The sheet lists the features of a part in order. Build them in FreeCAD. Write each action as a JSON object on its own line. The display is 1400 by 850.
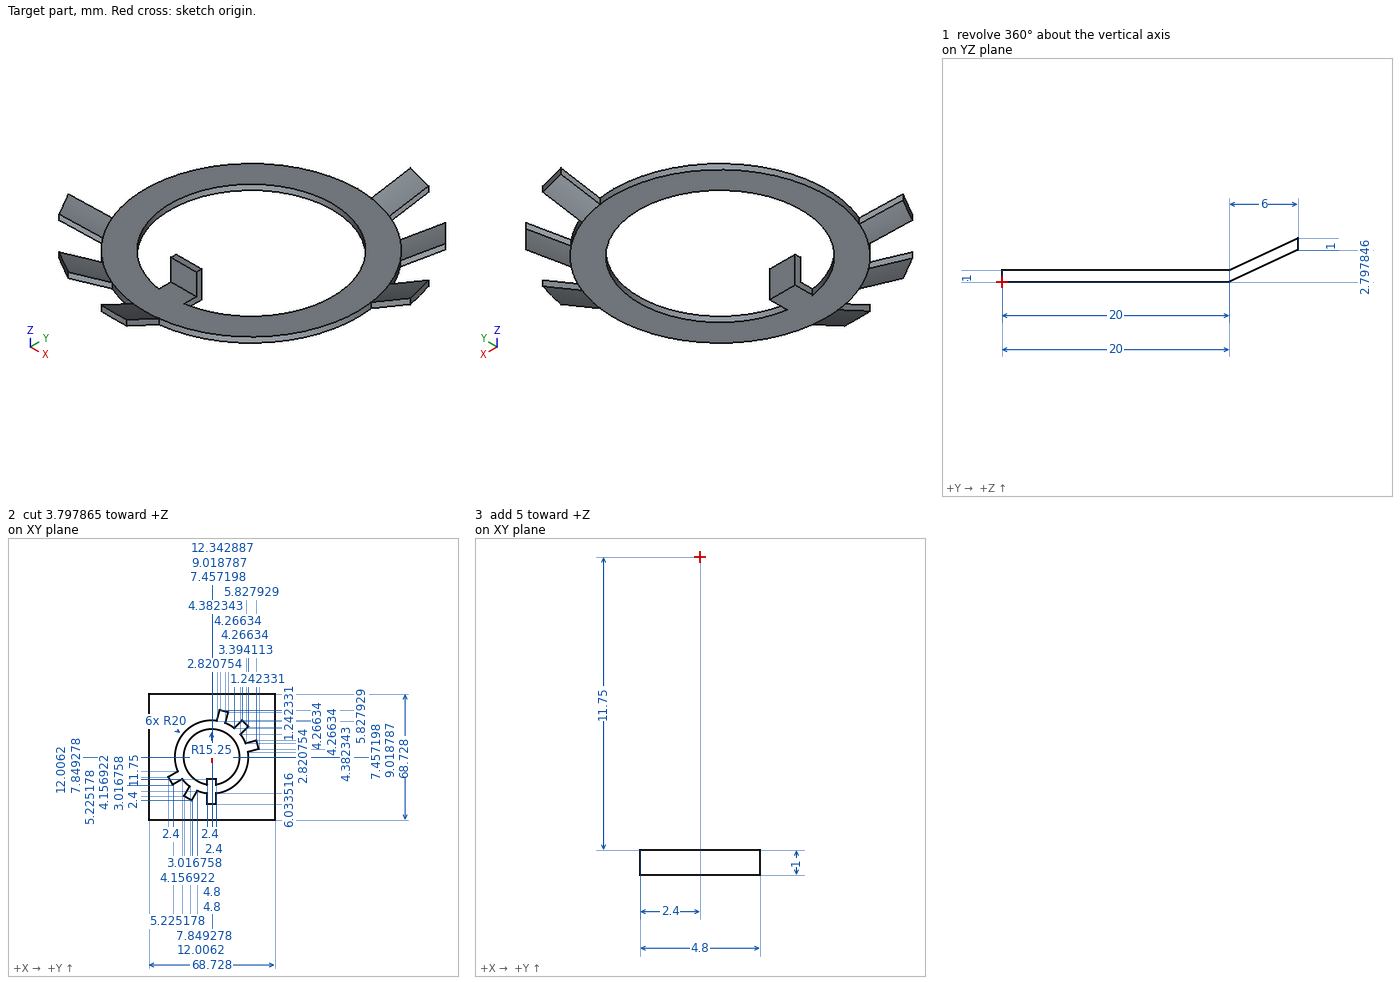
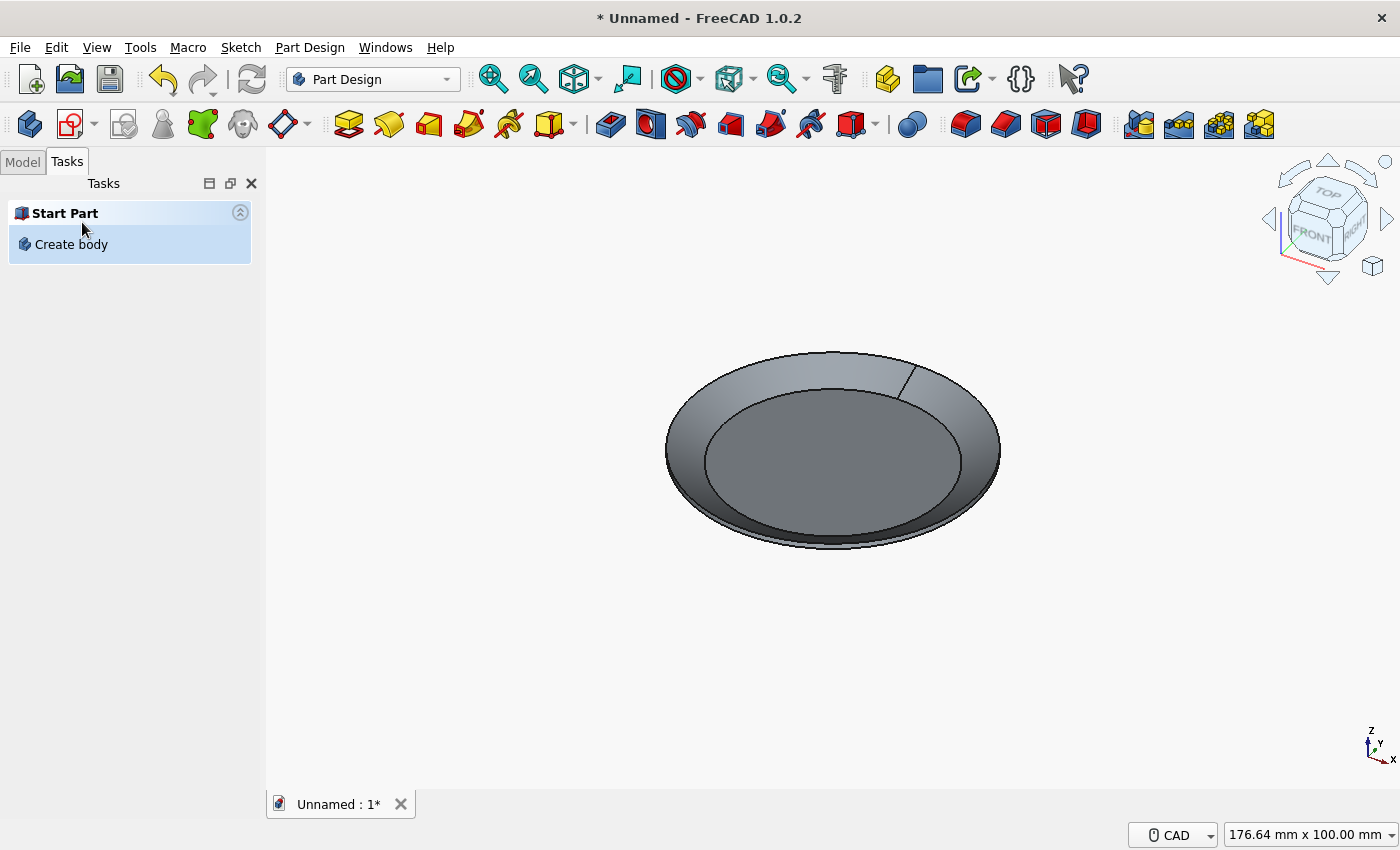
{"action": "left_click", "coordinate": [494, 80]}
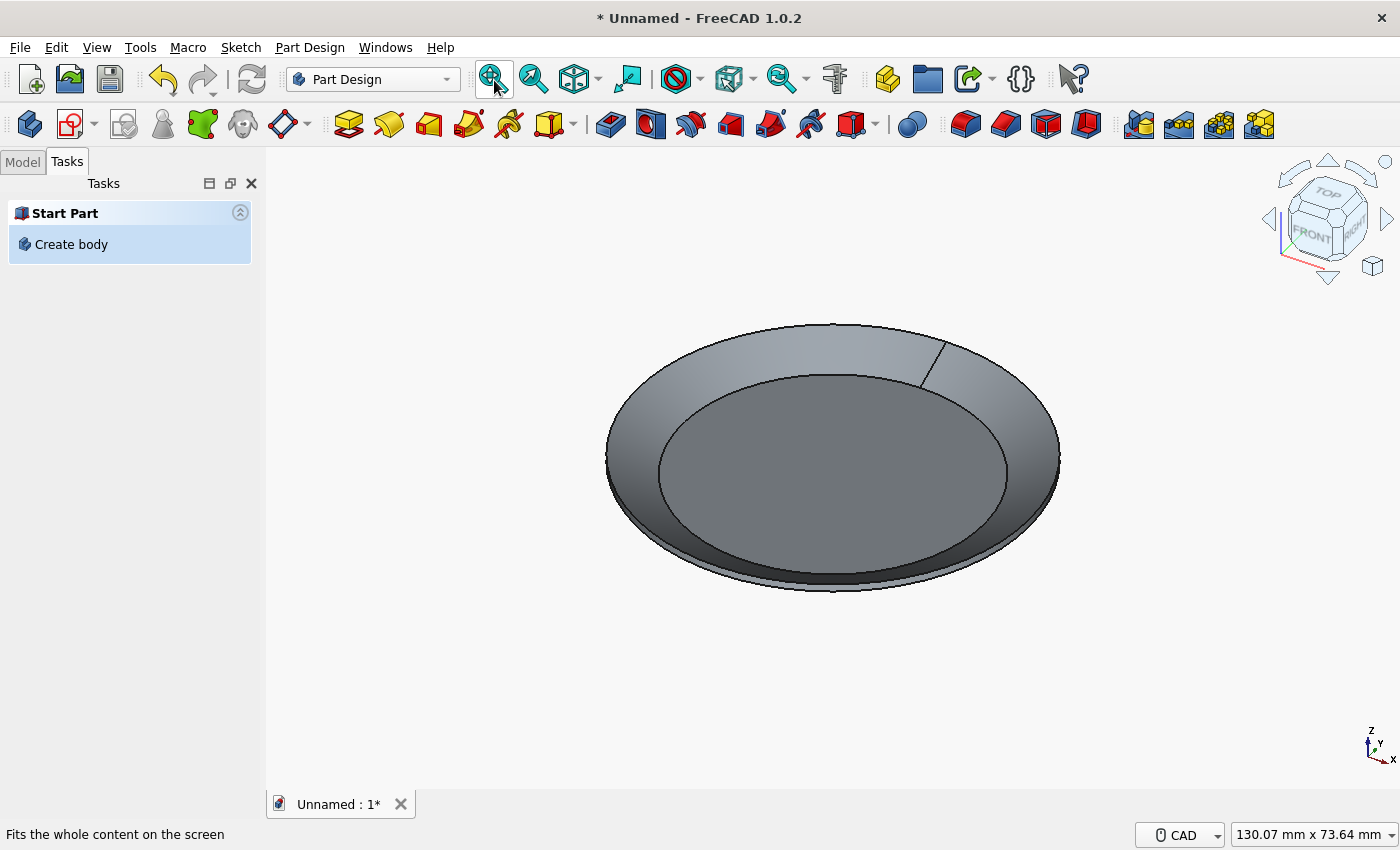
{"action": "left_click", "coordinate": [70, 124]}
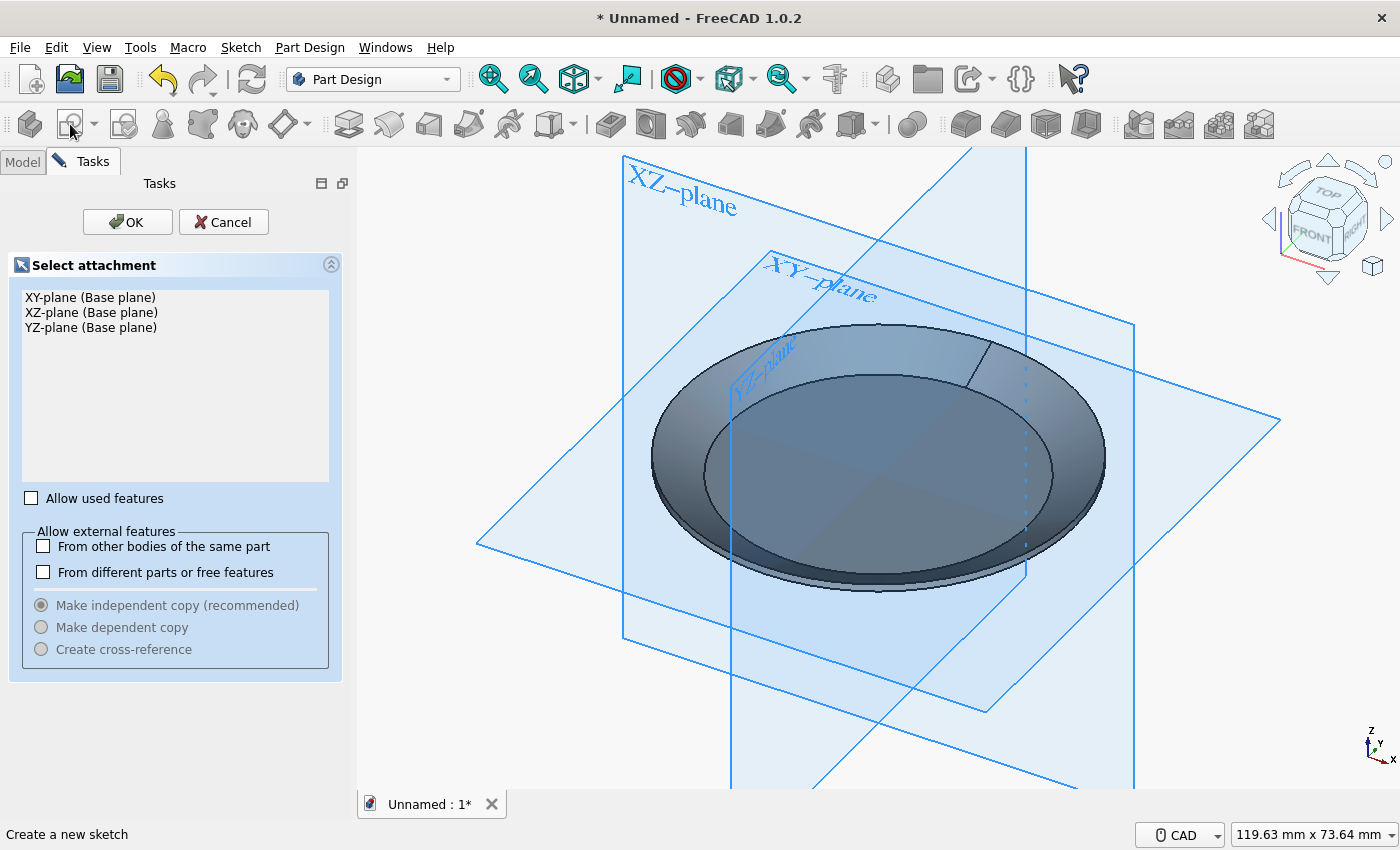
{"action": "left_click", "coordinate": [82, 298]}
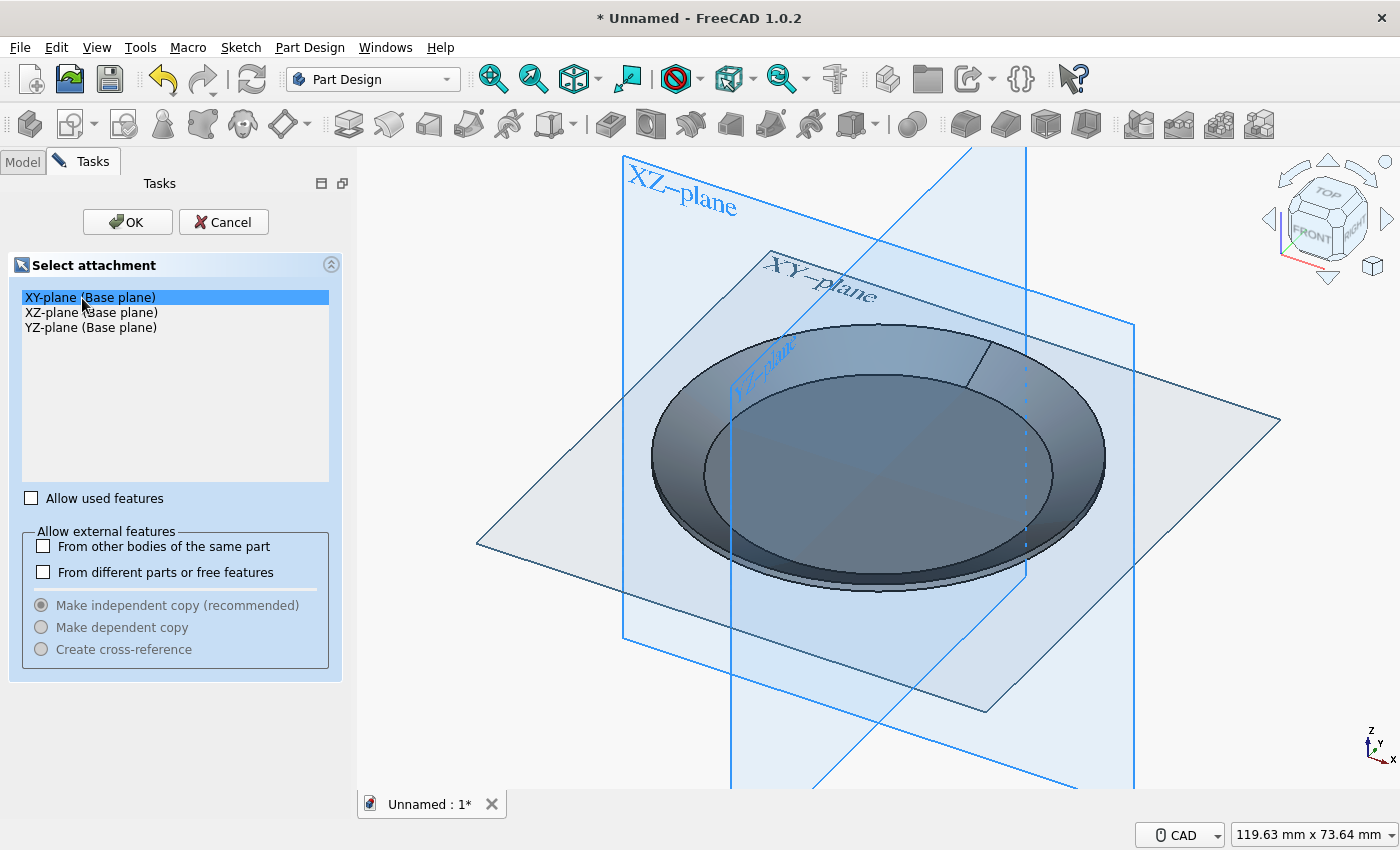
{"action": "left_click", "coordinate": [128, 222]}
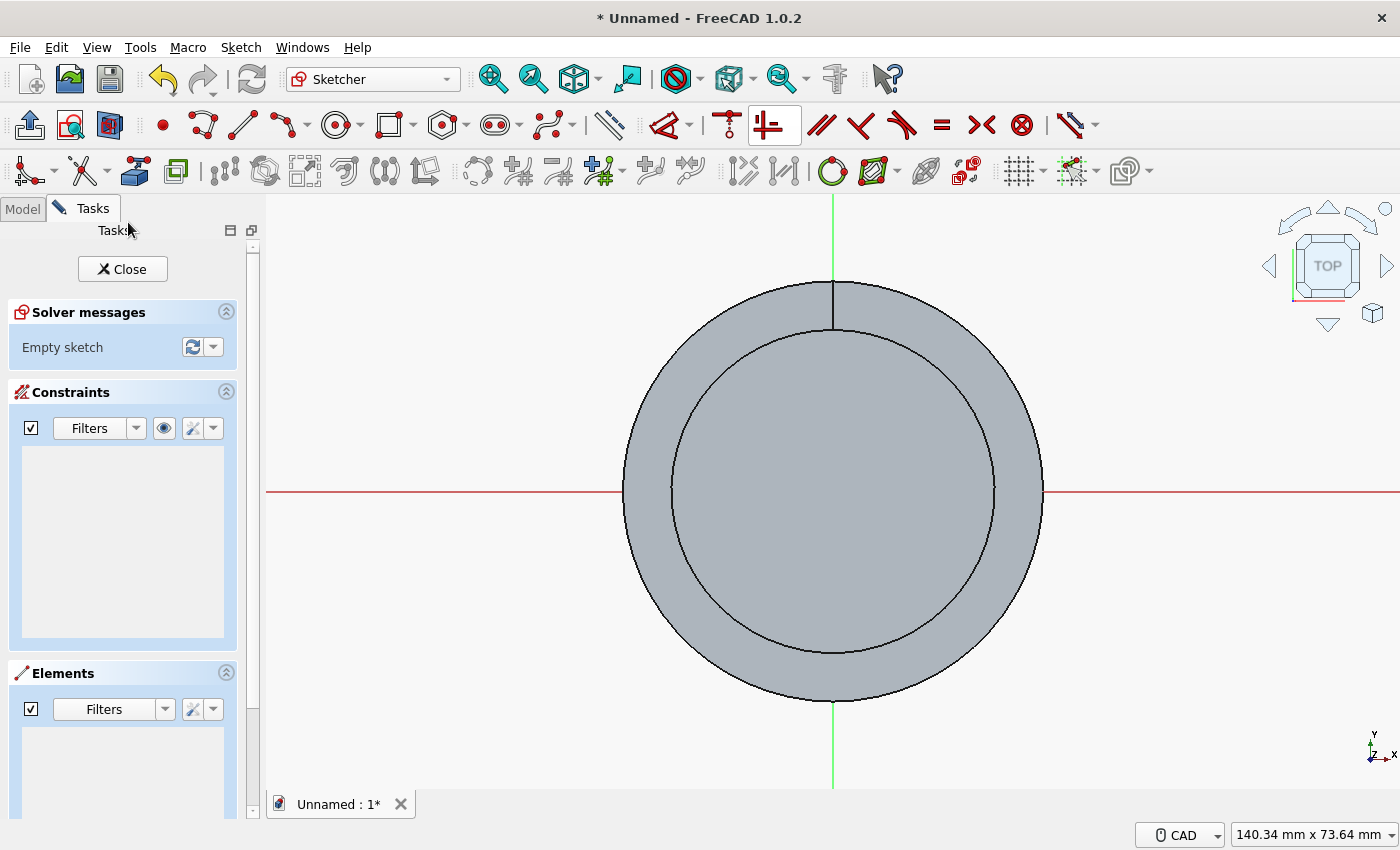
{"action": "left_click", "coordinate": [110, 126]}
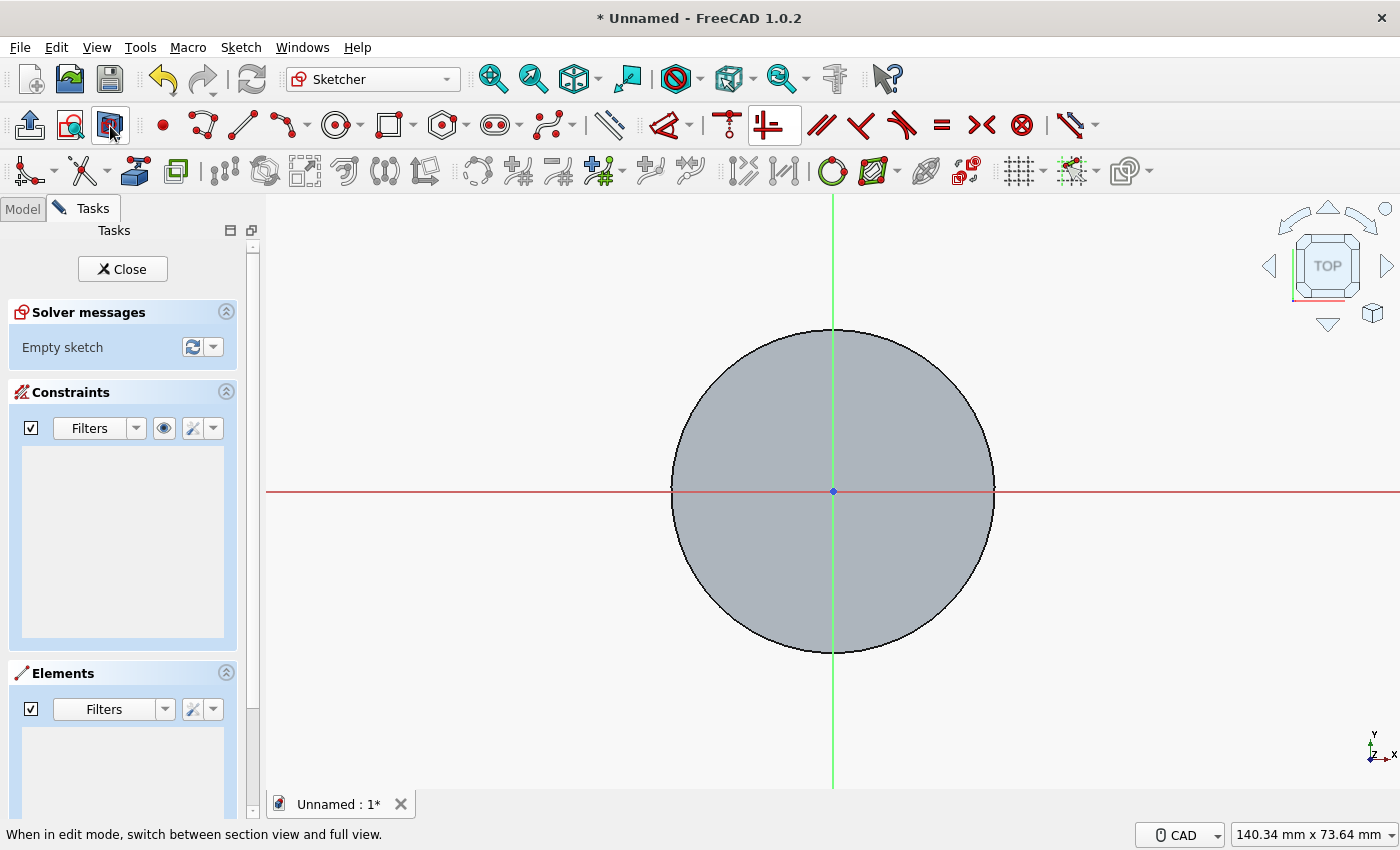
{"action": "scroll", "coordinate": [625, 492], "scroll_direction": "down", "scroll_amount": 2}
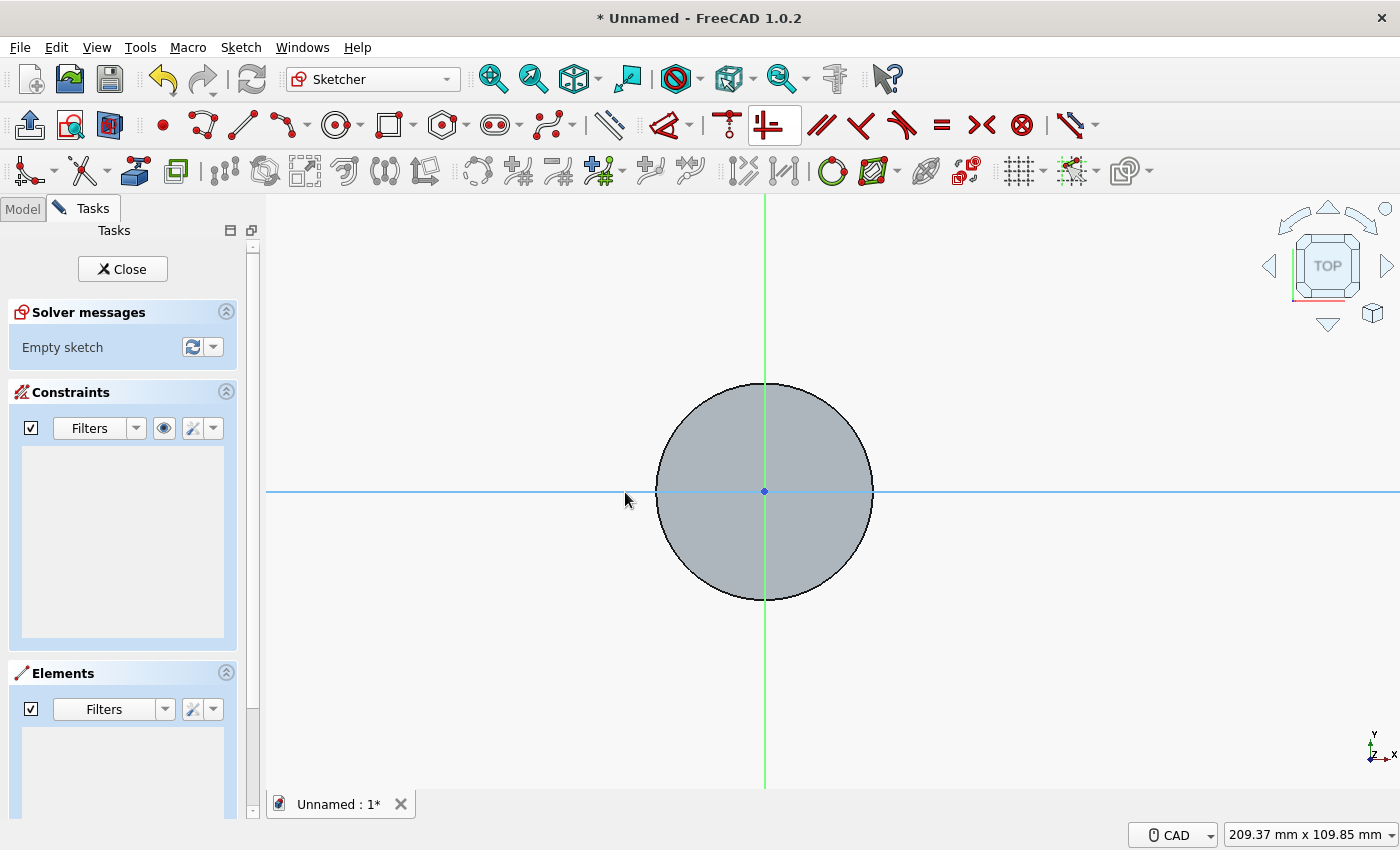
{"action": "left_click", "coordinate": [416, 126]}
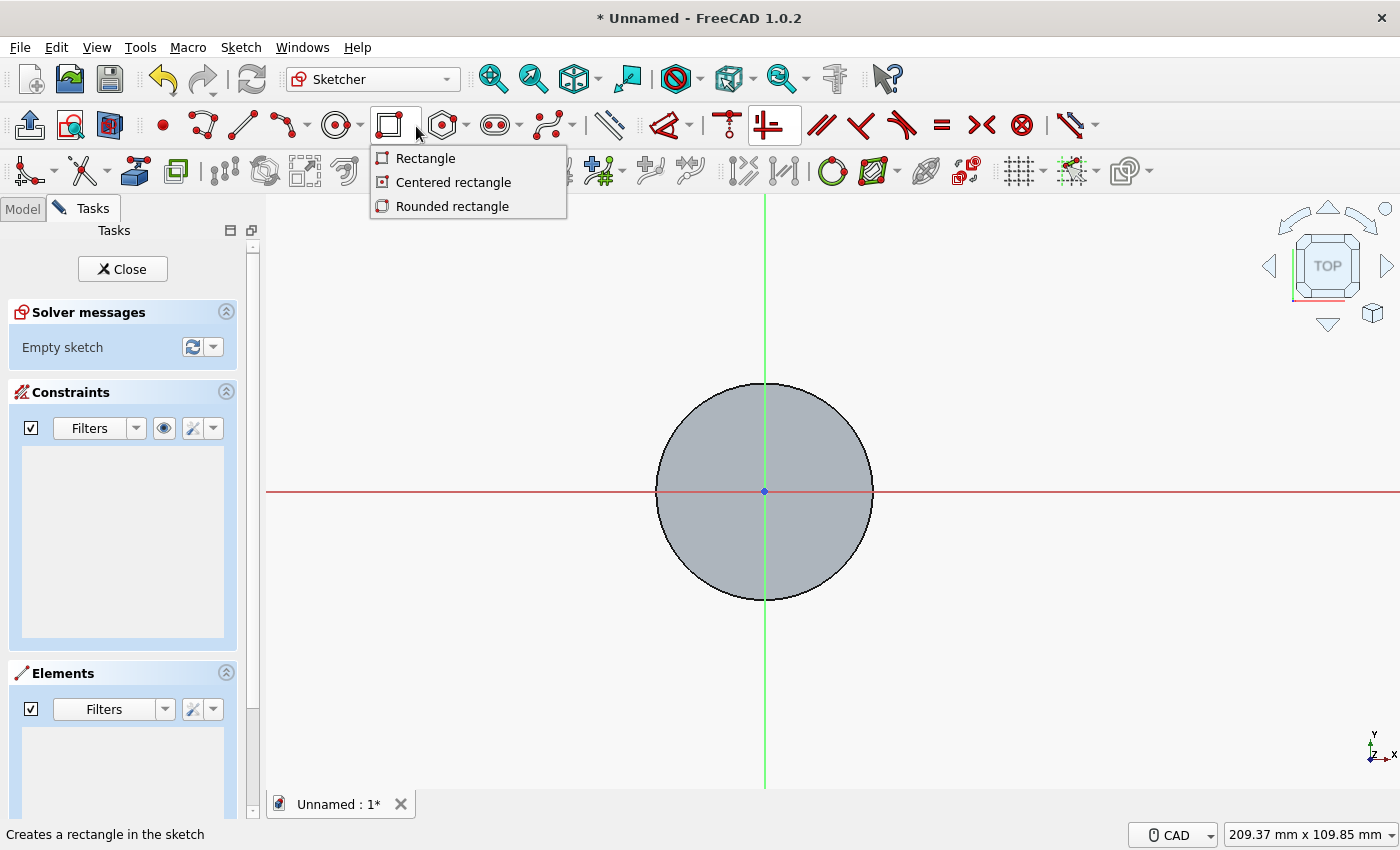
{"action": "left_click", "coordinate": [468, 182]}